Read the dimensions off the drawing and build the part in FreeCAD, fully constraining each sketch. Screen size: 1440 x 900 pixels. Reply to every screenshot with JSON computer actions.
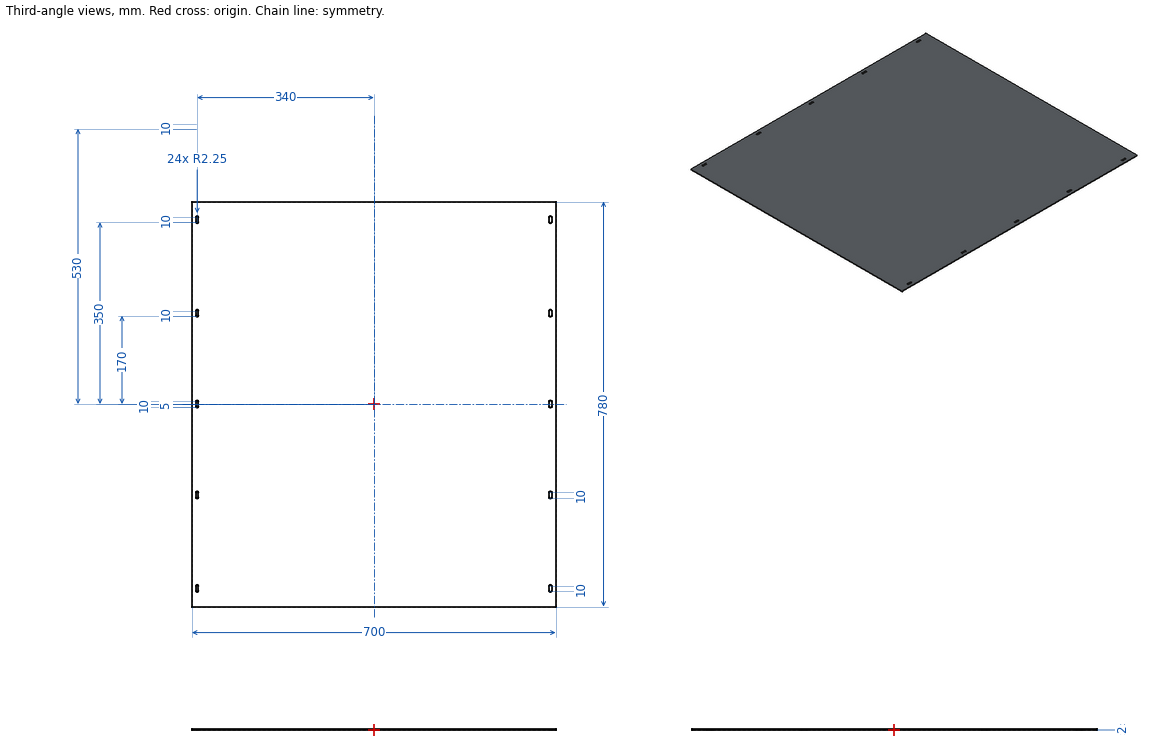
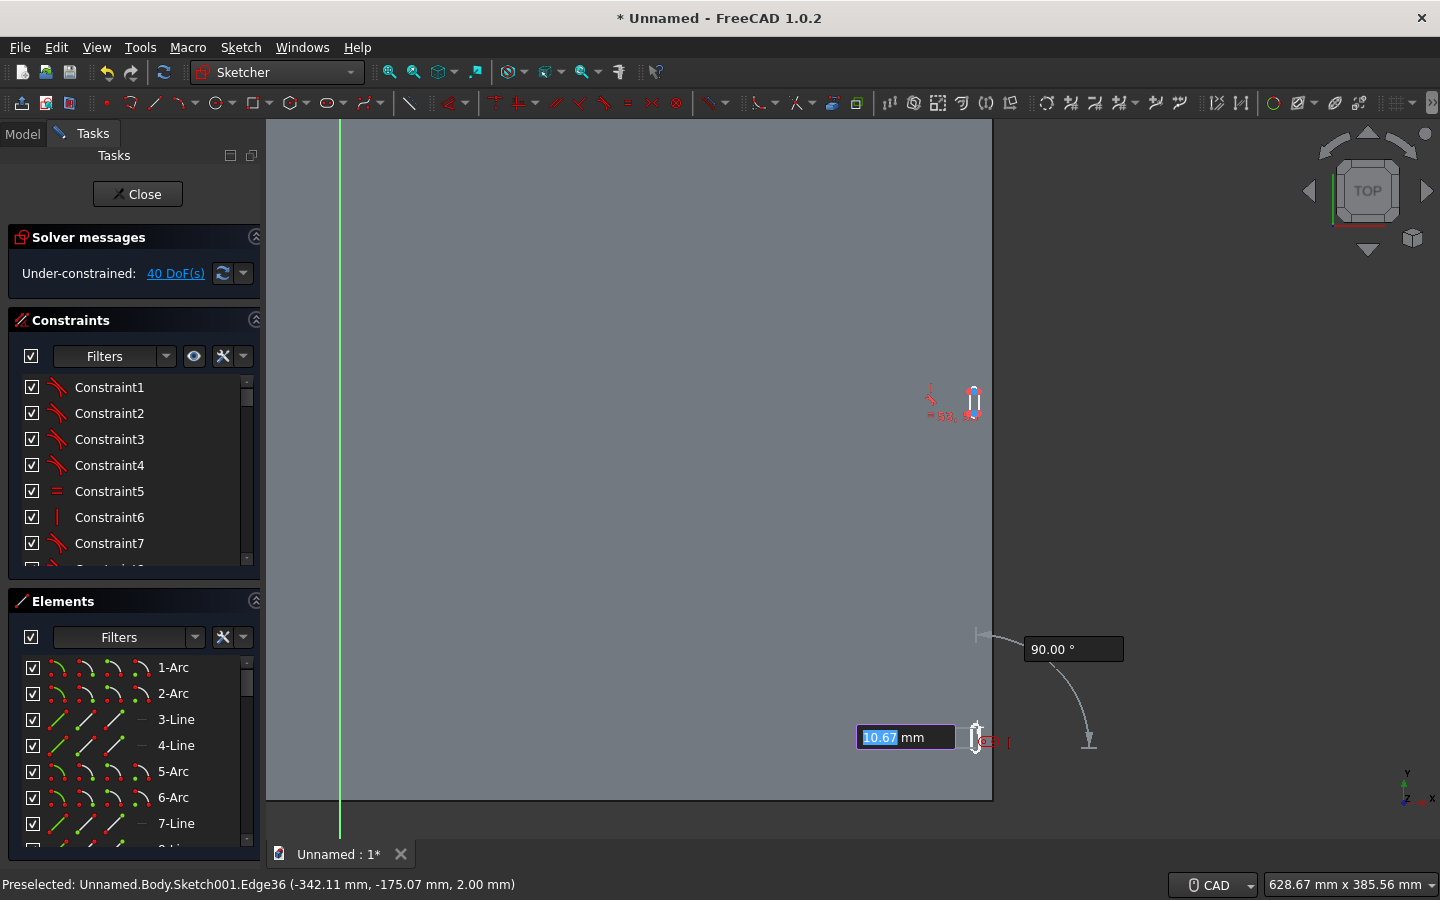
{"action": "left_click", "coordinate": [976, 727]}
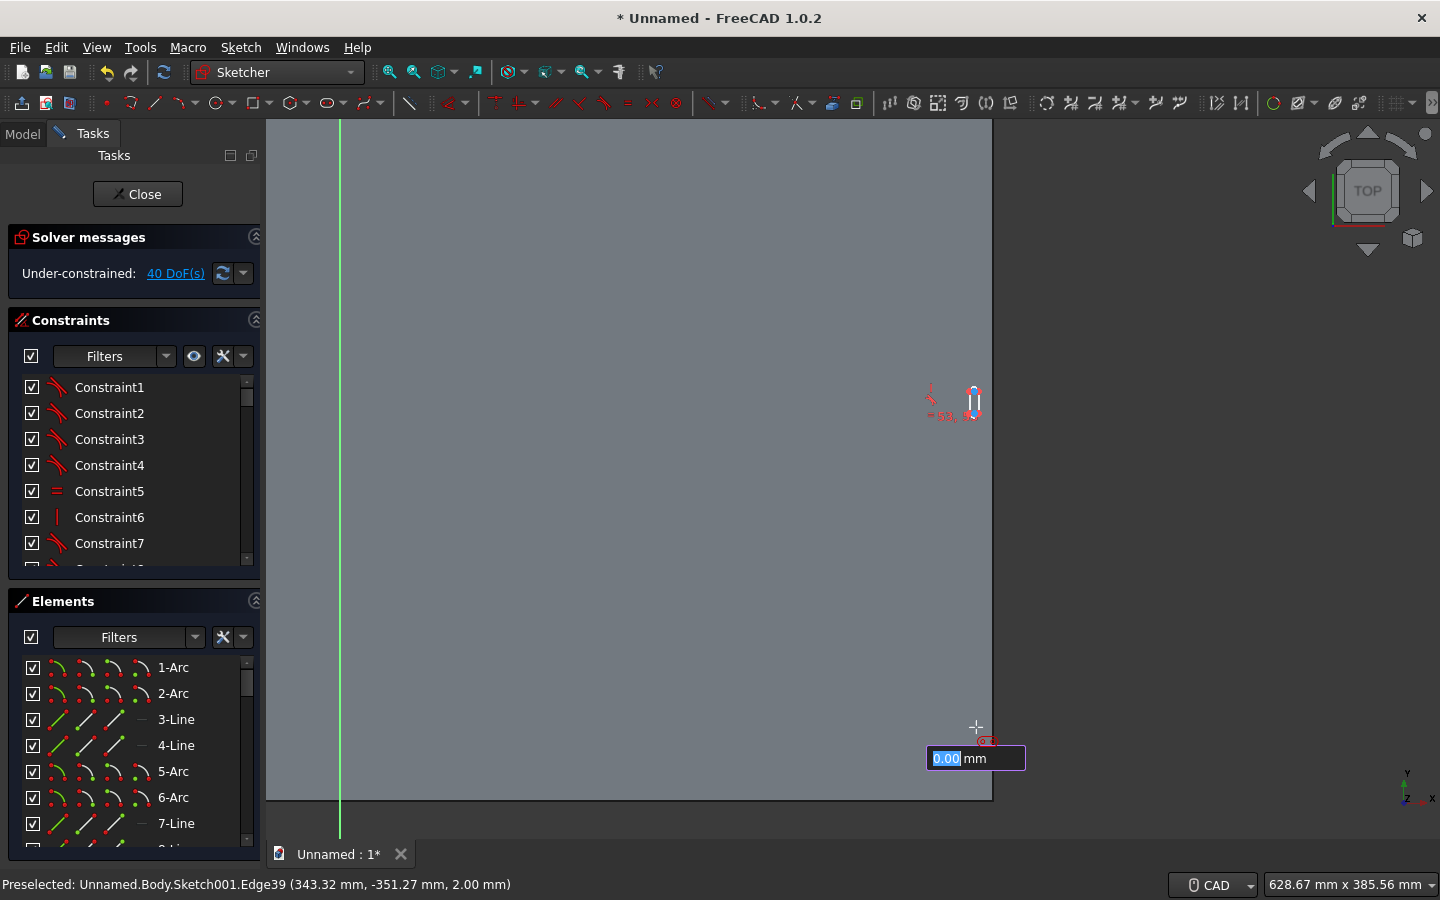
{"action": "scroll", "coordinate": [970, 736], "scroll_direction": "up", "scroll_amount": 7}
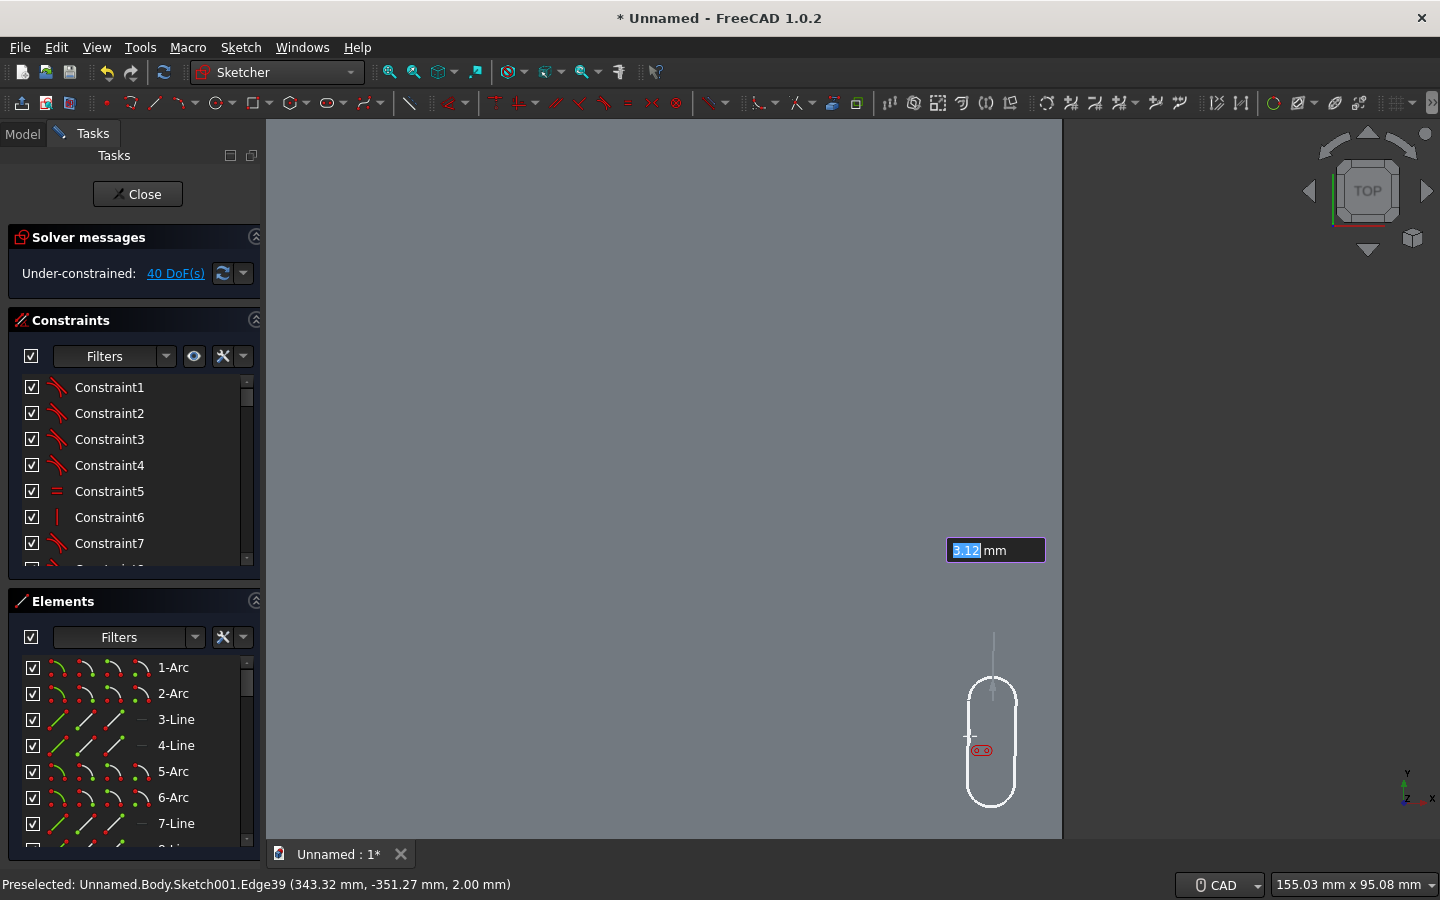
{"action": "left_click", "coordinate": [970, 733]}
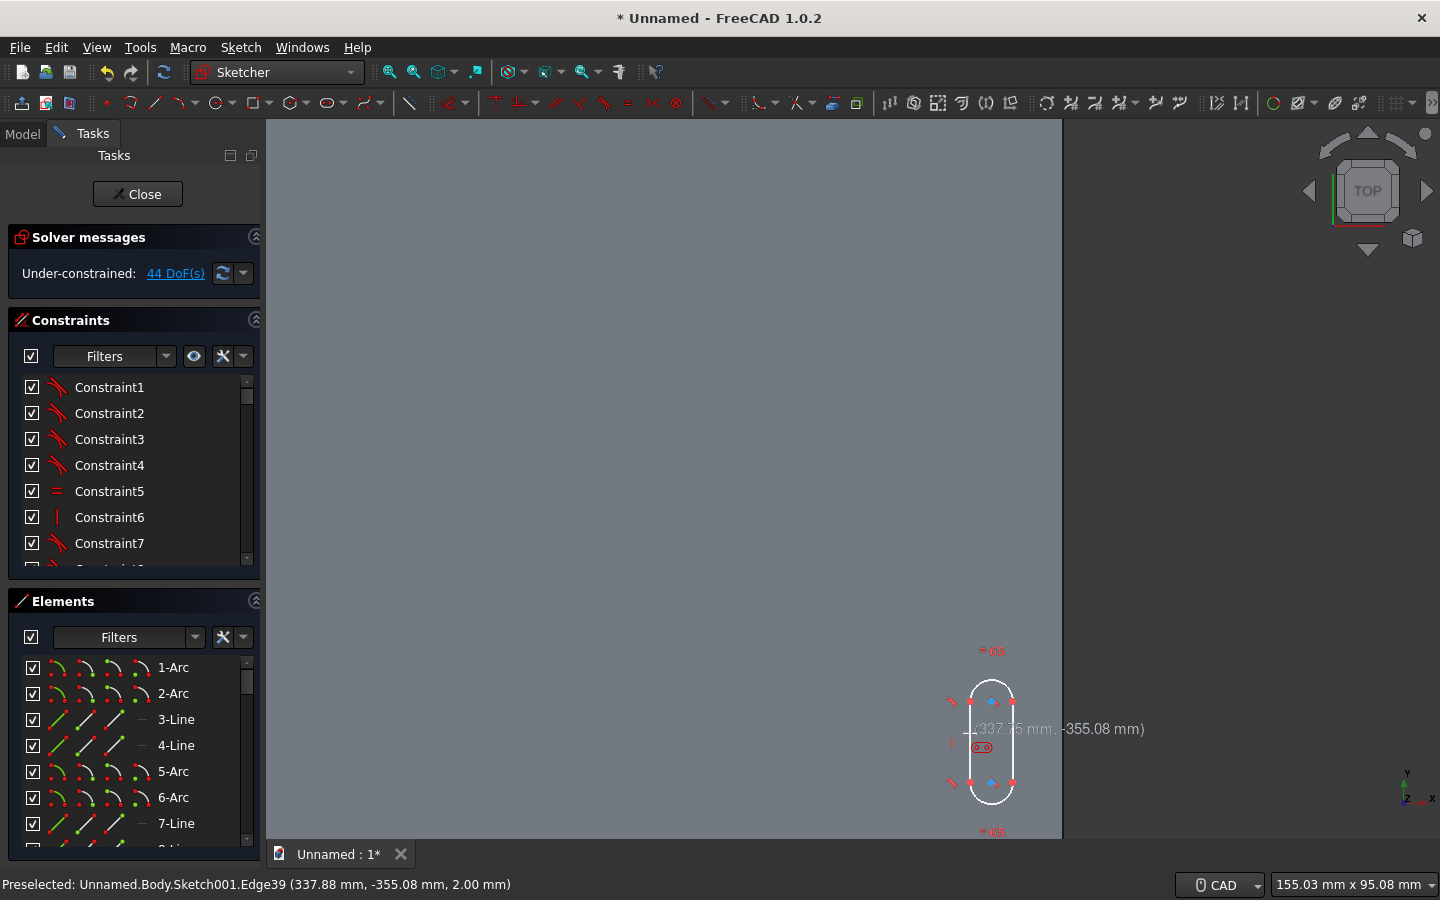
{"action": "scroll", "coordinate": [975, 729], "scroll_direction": "down", "scroll_amount": 13}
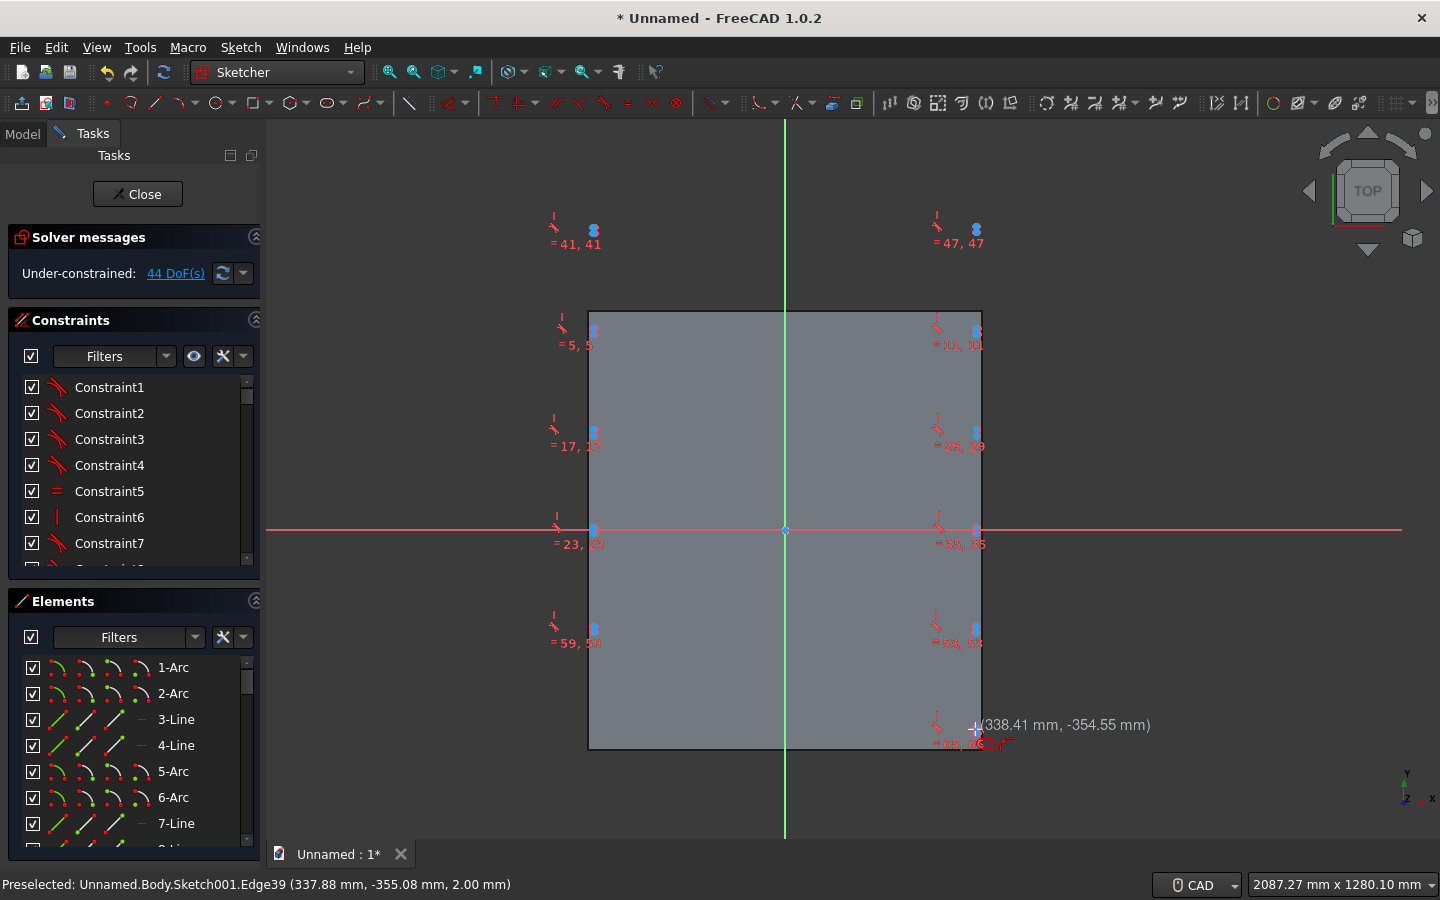
{"action": "scroll", "coordinate": [594, 733], "scroll_direction": "up", "scroll_amount": 15}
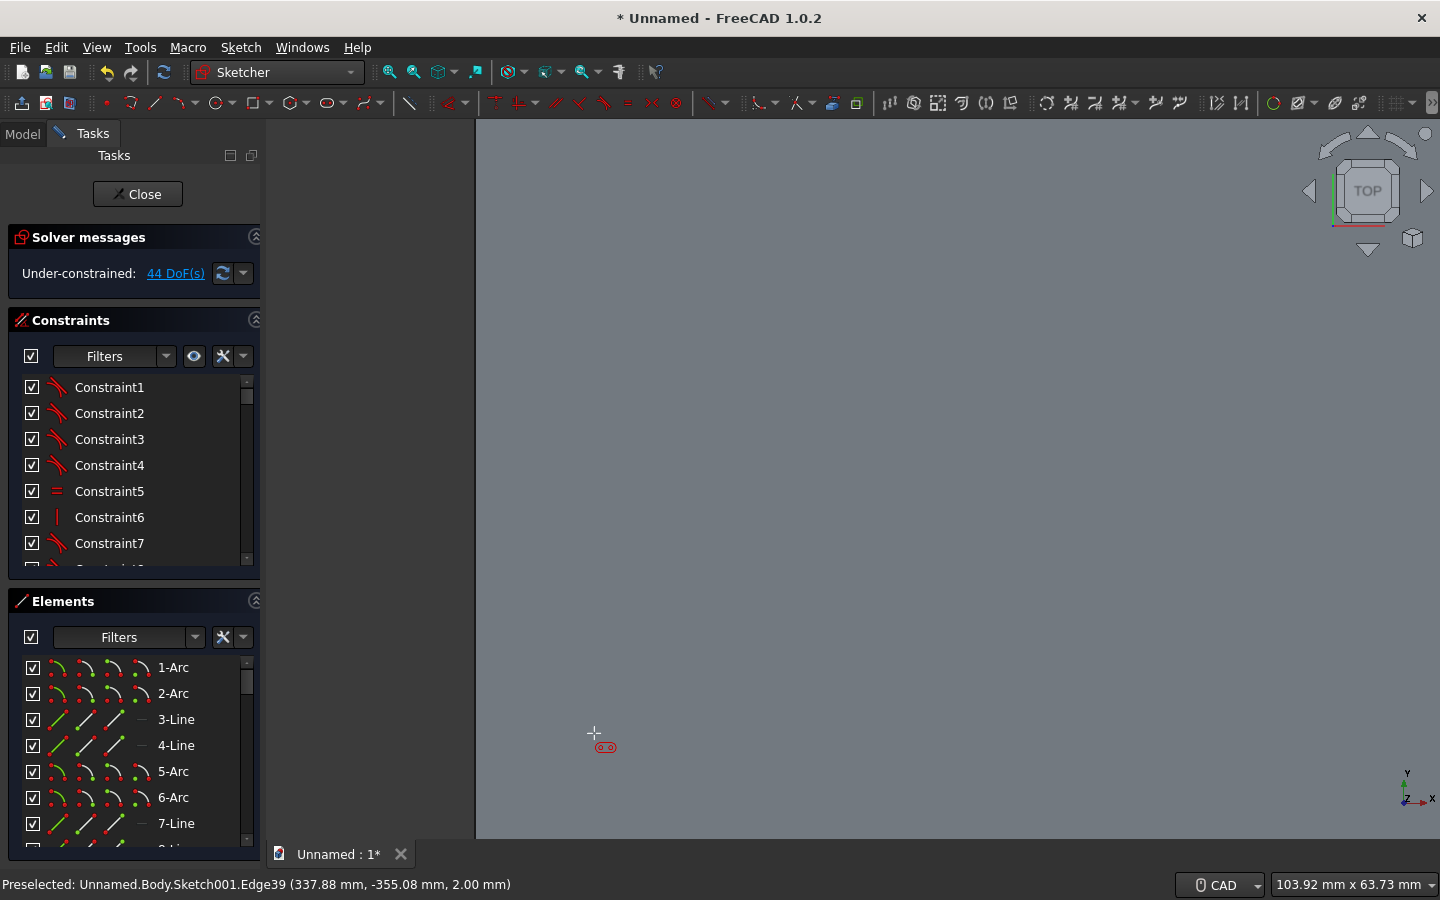
{"action": "scroll", "coordinate": [594, 733], "scroll_direction": "down", "scroll_amount": 15}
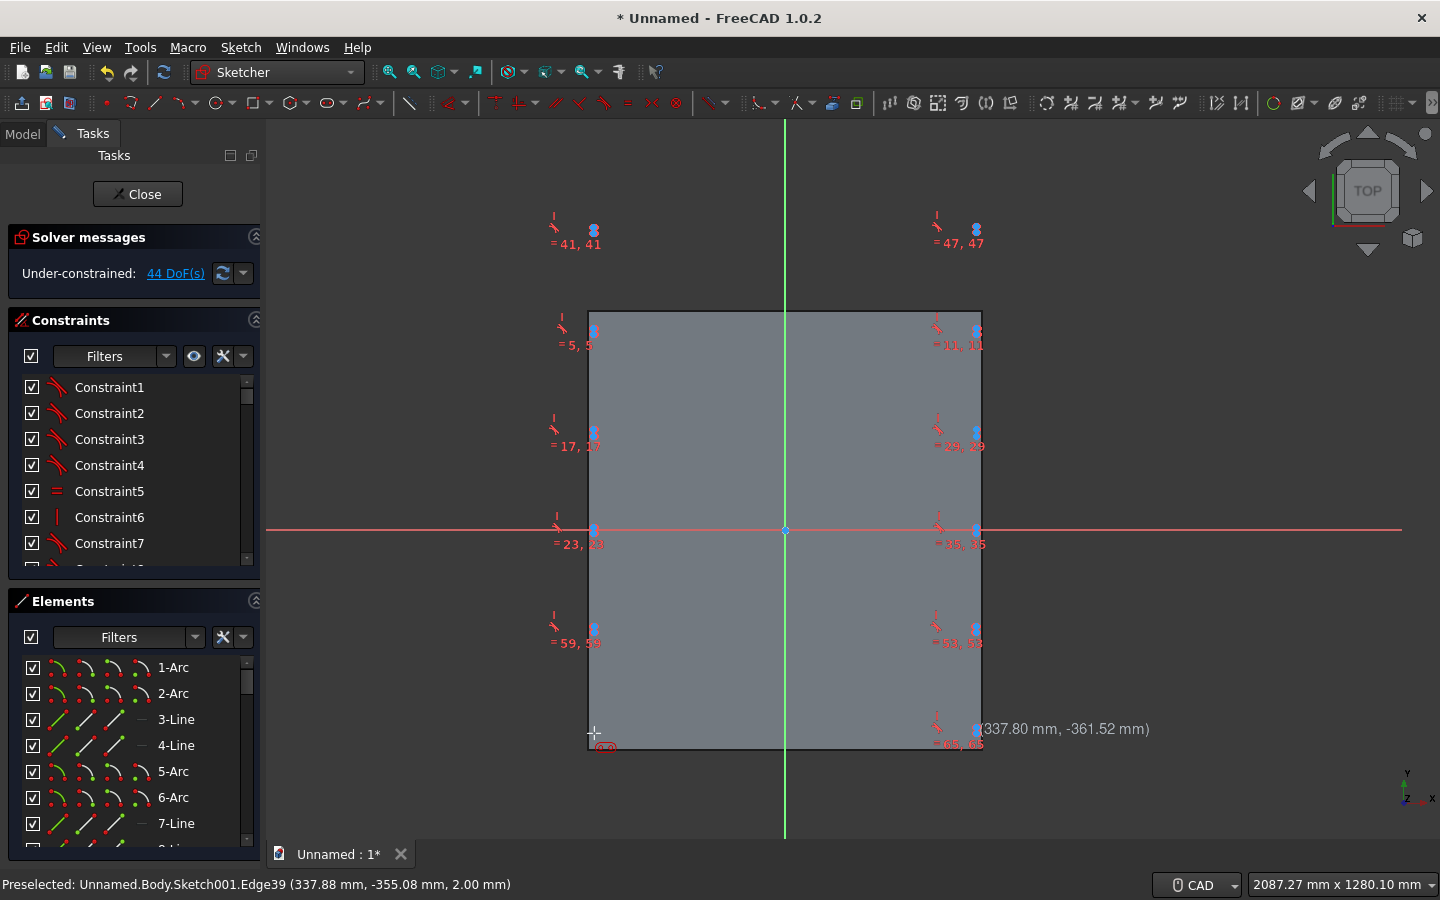
{"action": "left_click", "coordinate": [594, 733]}